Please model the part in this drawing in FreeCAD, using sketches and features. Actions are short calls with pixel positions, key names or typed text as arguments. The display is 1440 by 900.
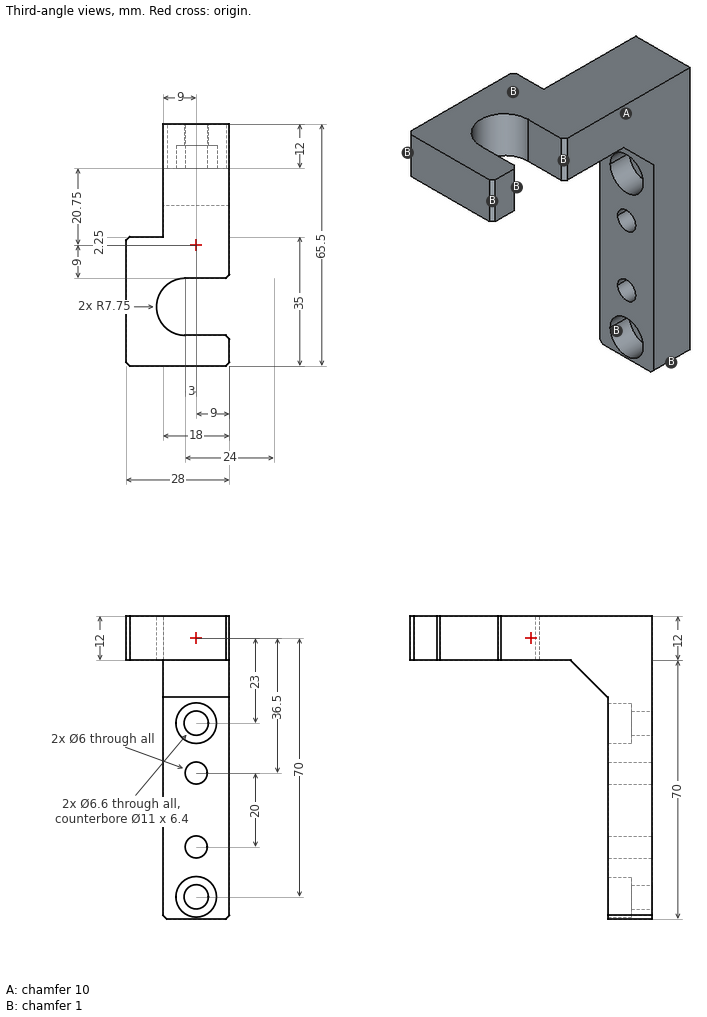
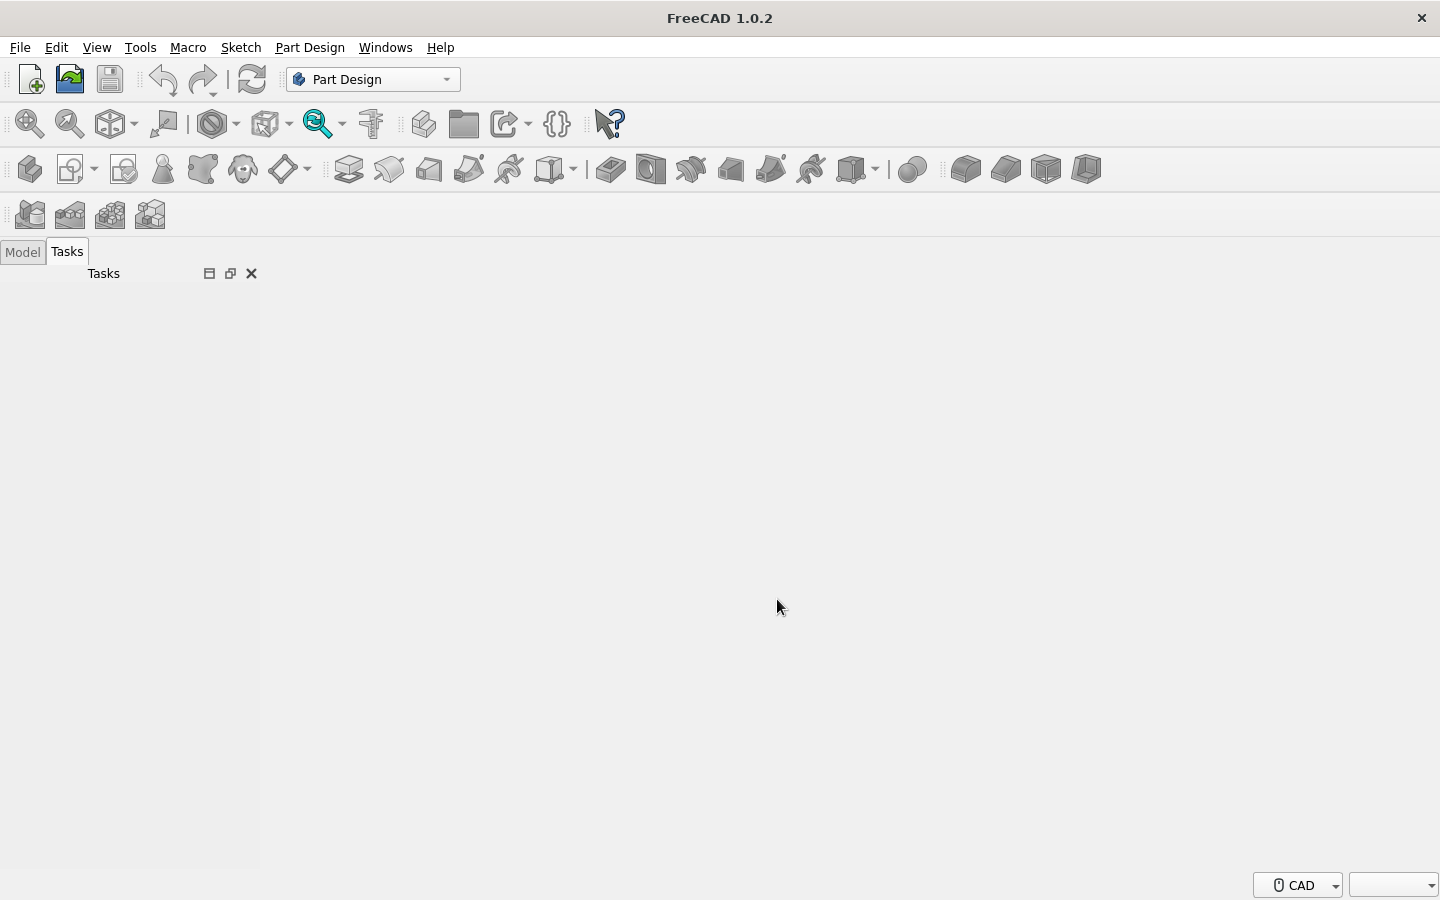
key(ctrl+n)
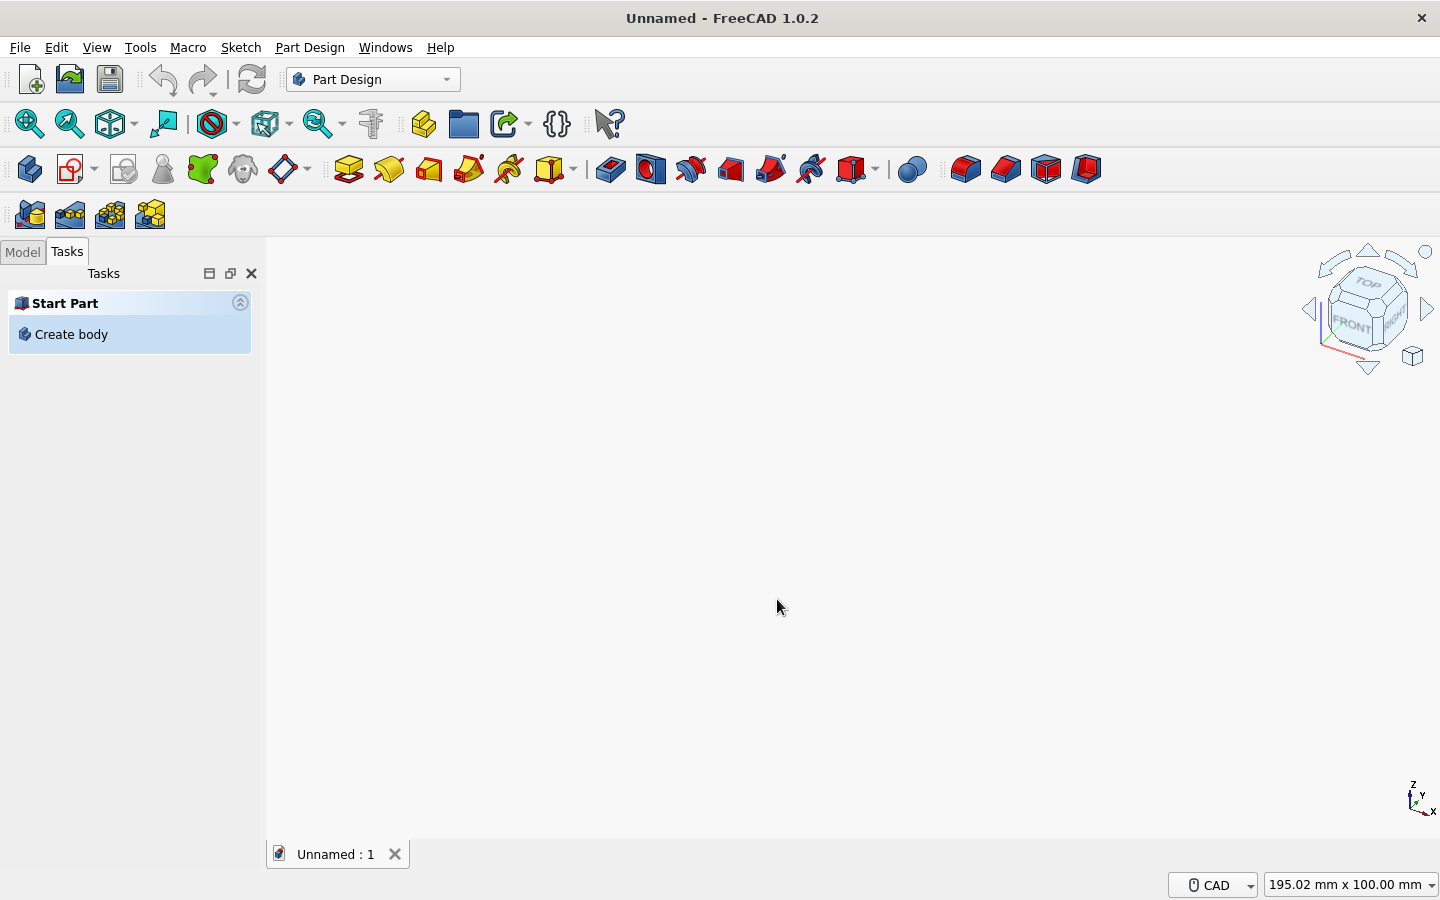
click(70, 170)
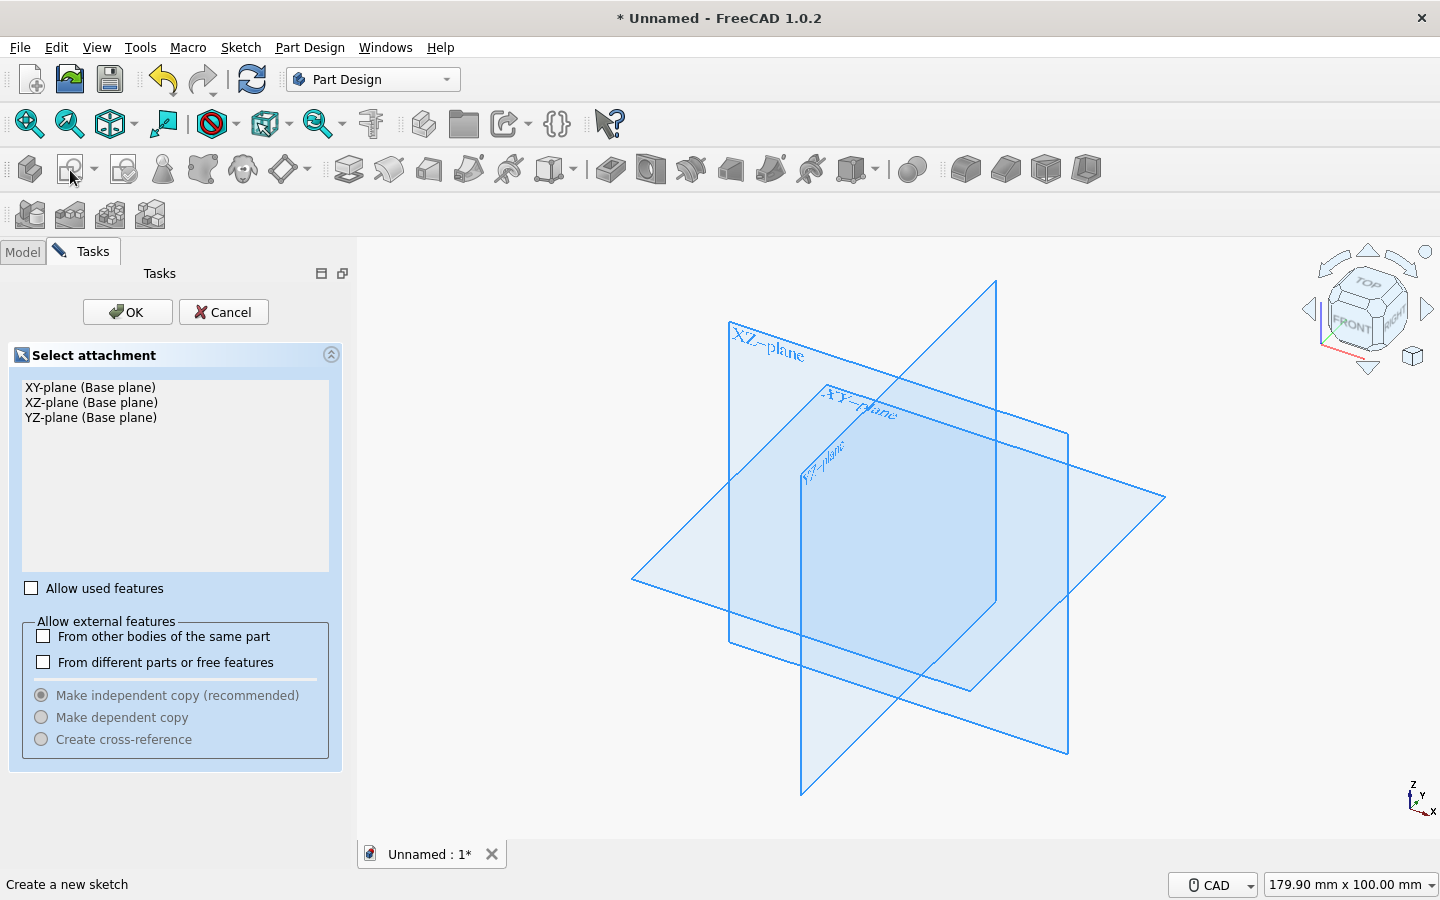
click(82, 388)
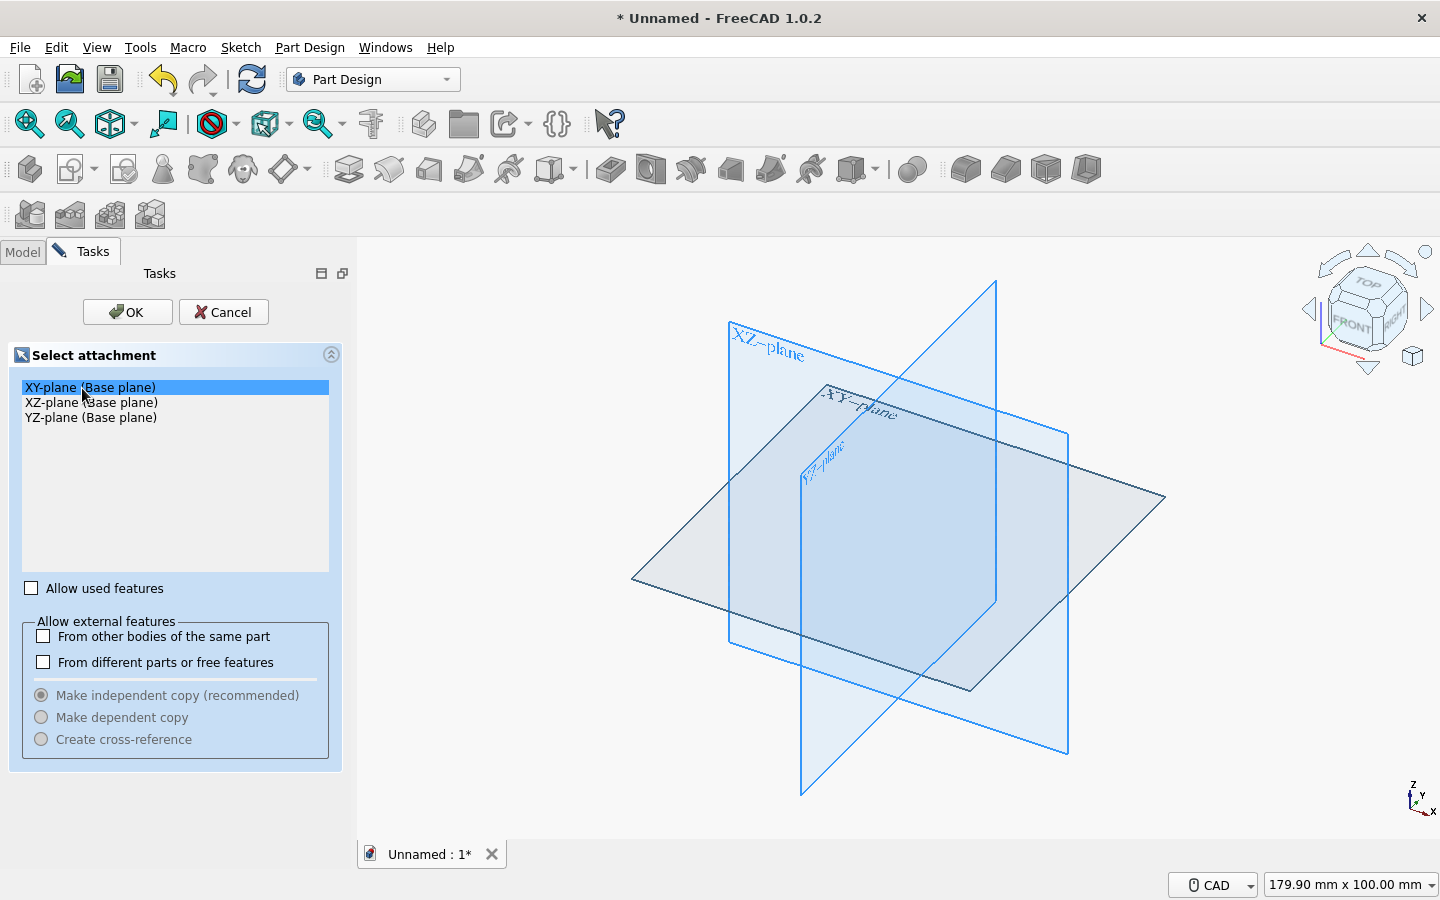
click(128, 312)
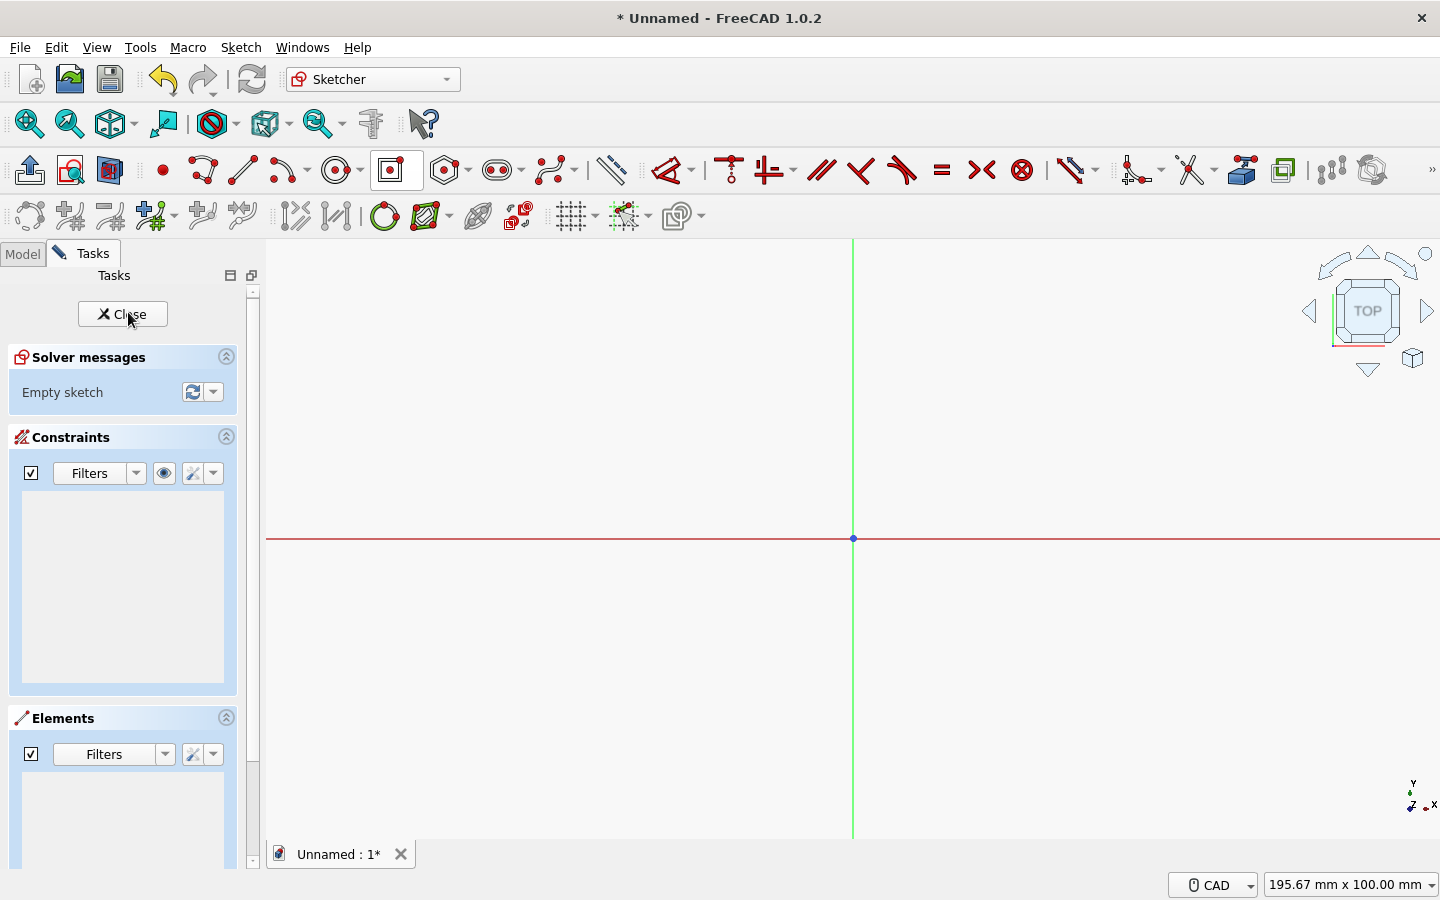
click(390, 170)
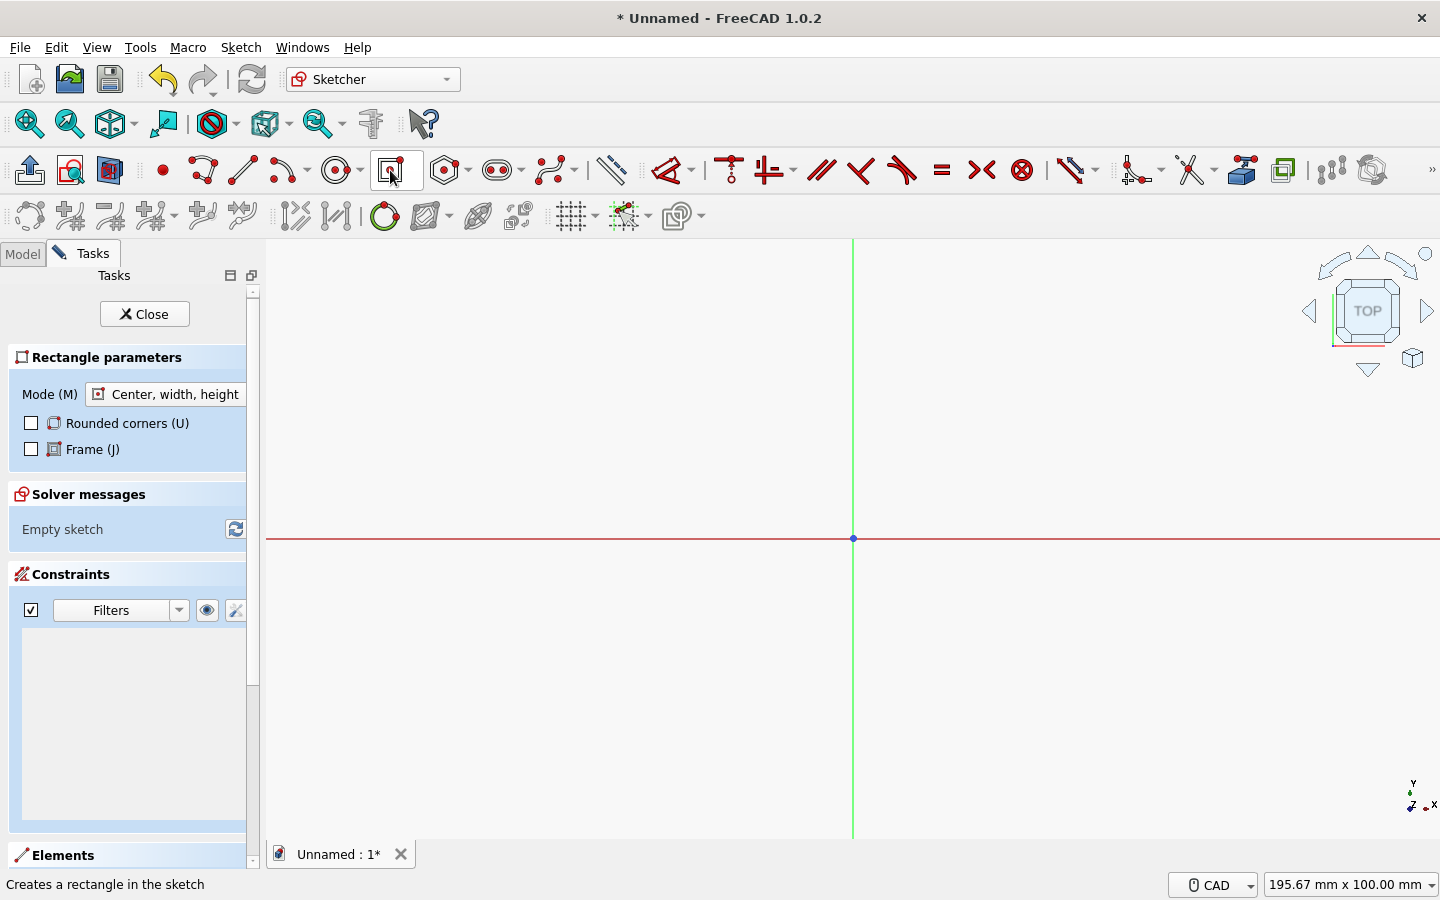
click(853, 539)
move(907, 342)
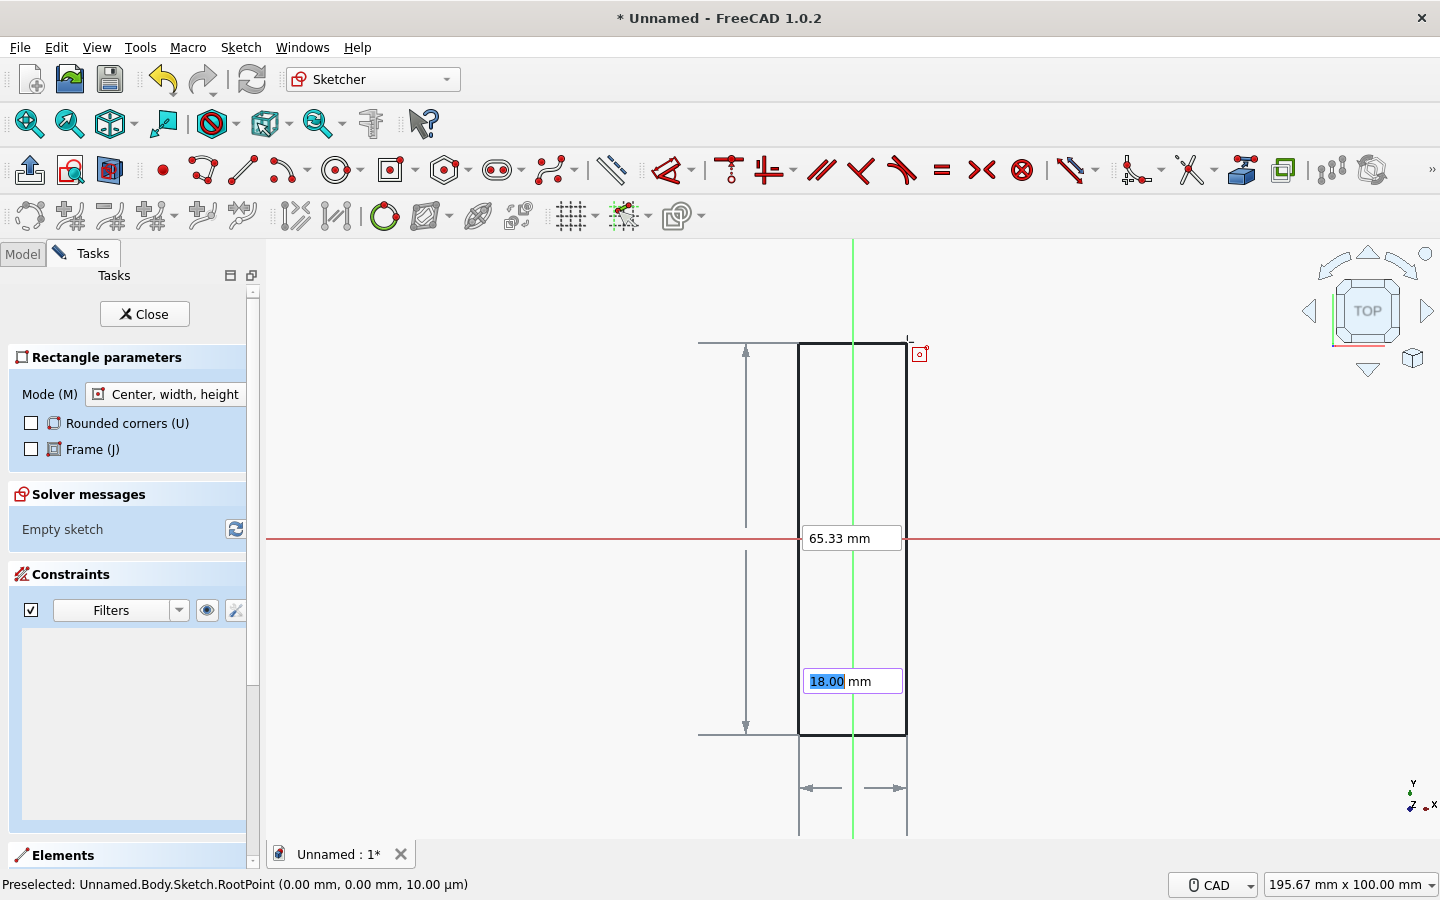
text(18)
key(Tab)
text(65.5)
key(Return)
key(Escape)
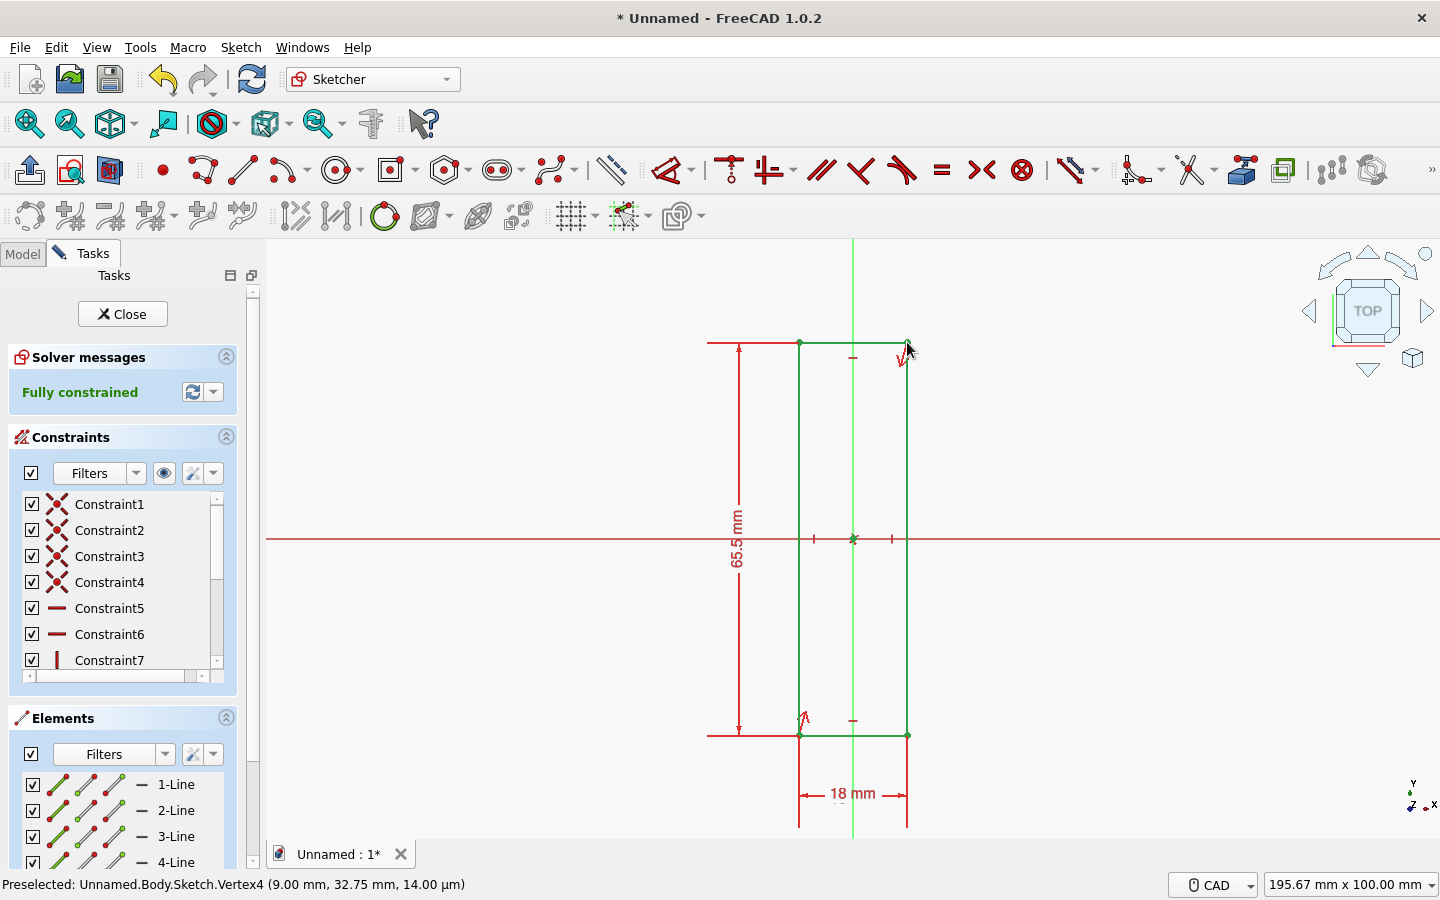
click(123, 314)